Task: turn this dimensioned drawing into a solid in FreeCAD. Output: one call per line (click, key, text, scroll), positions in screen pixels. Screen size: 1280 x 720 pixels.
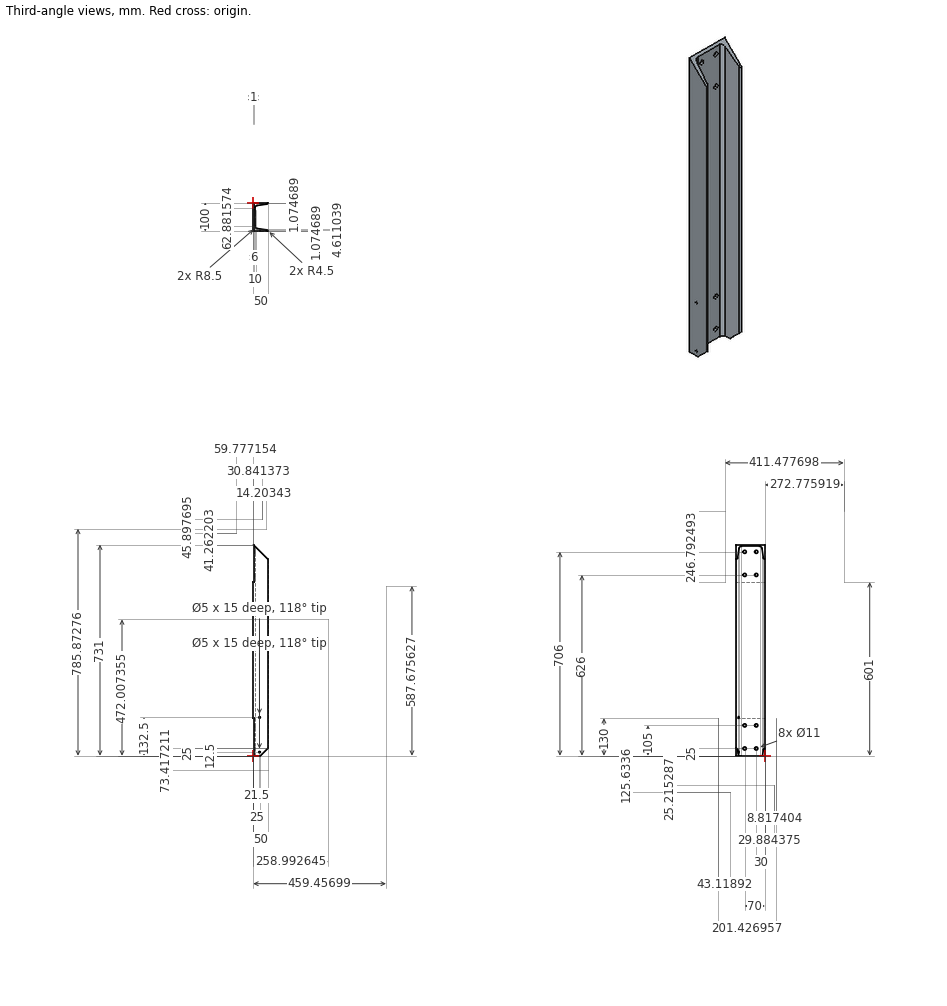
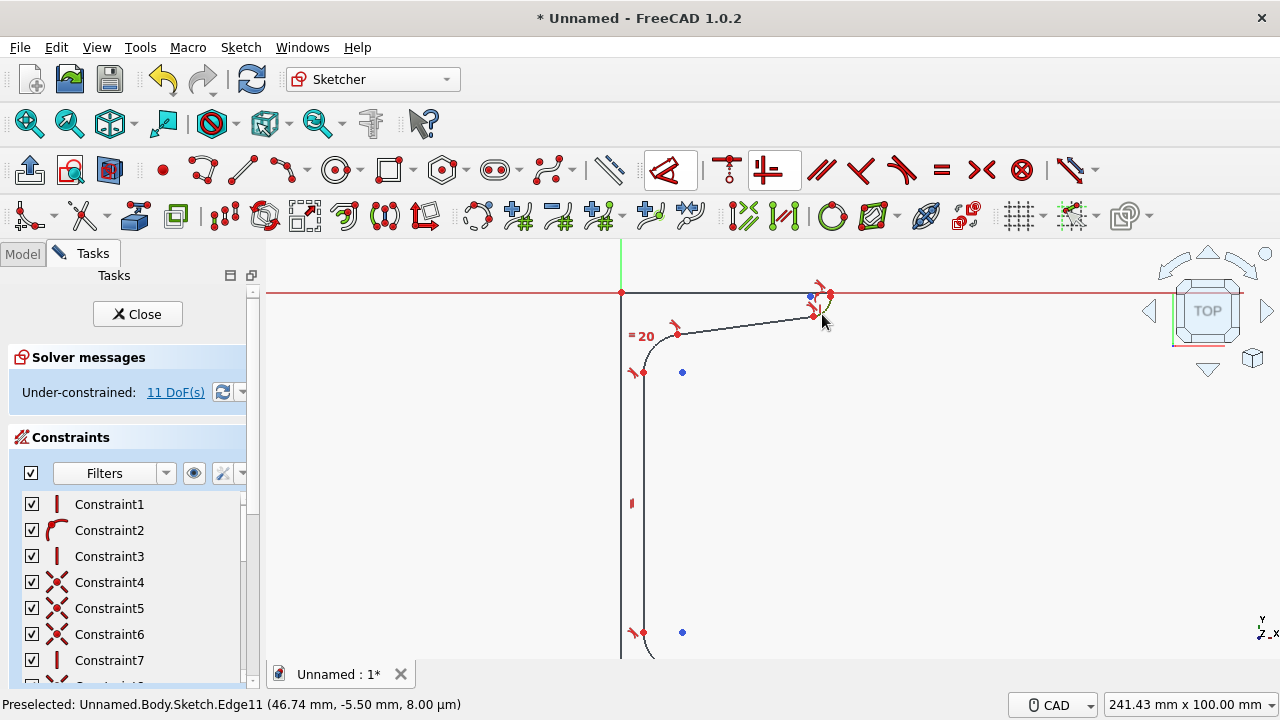
scroll(661, 340, down, 2)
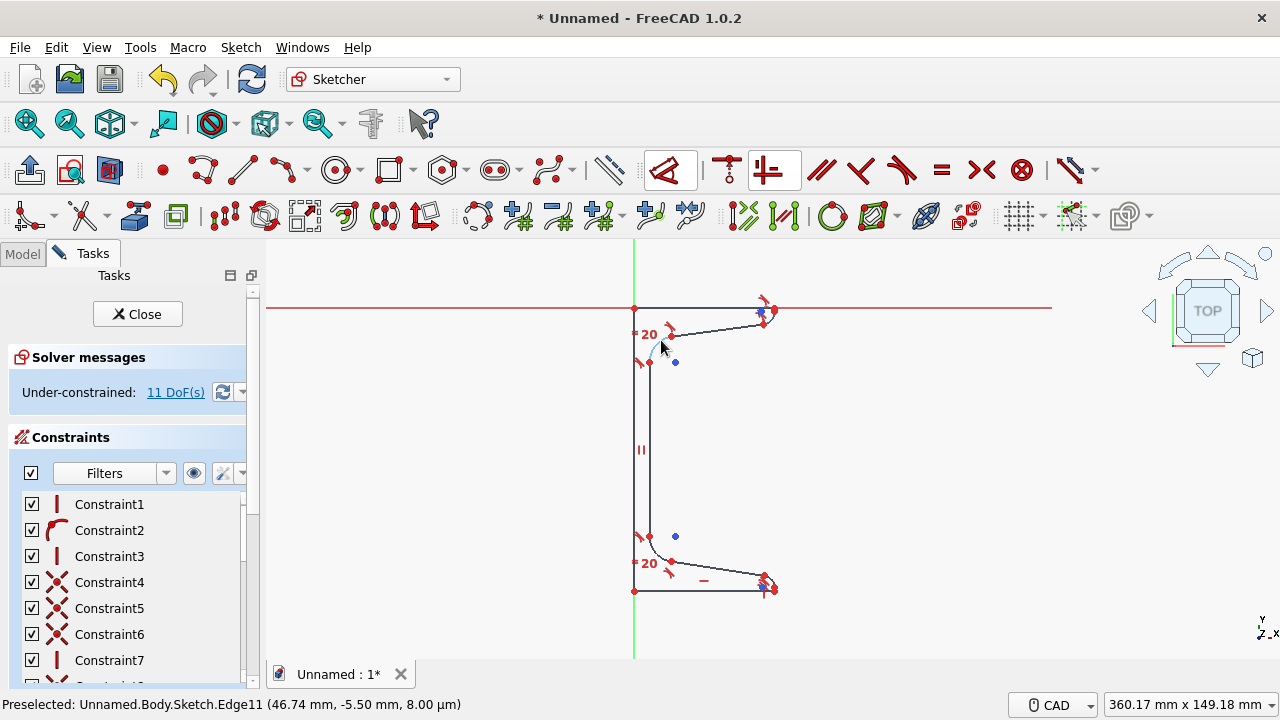
scroll(772, 580, up, 3)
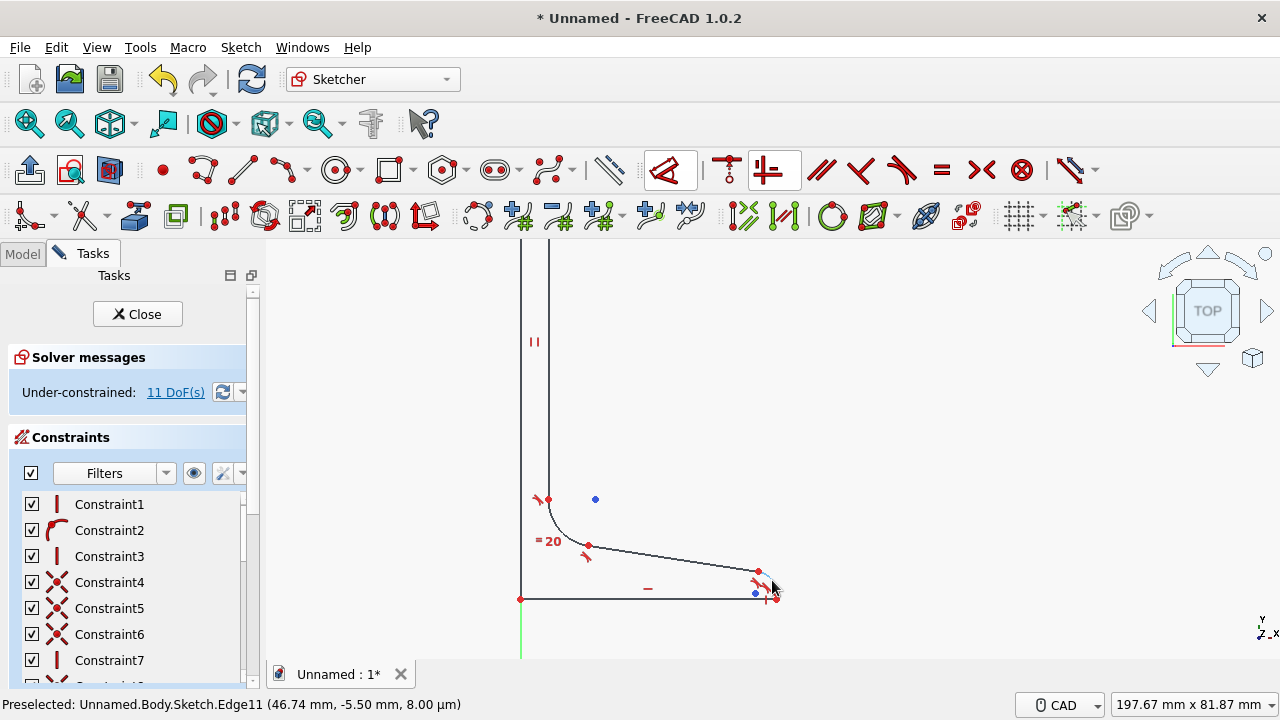
click(771, 579)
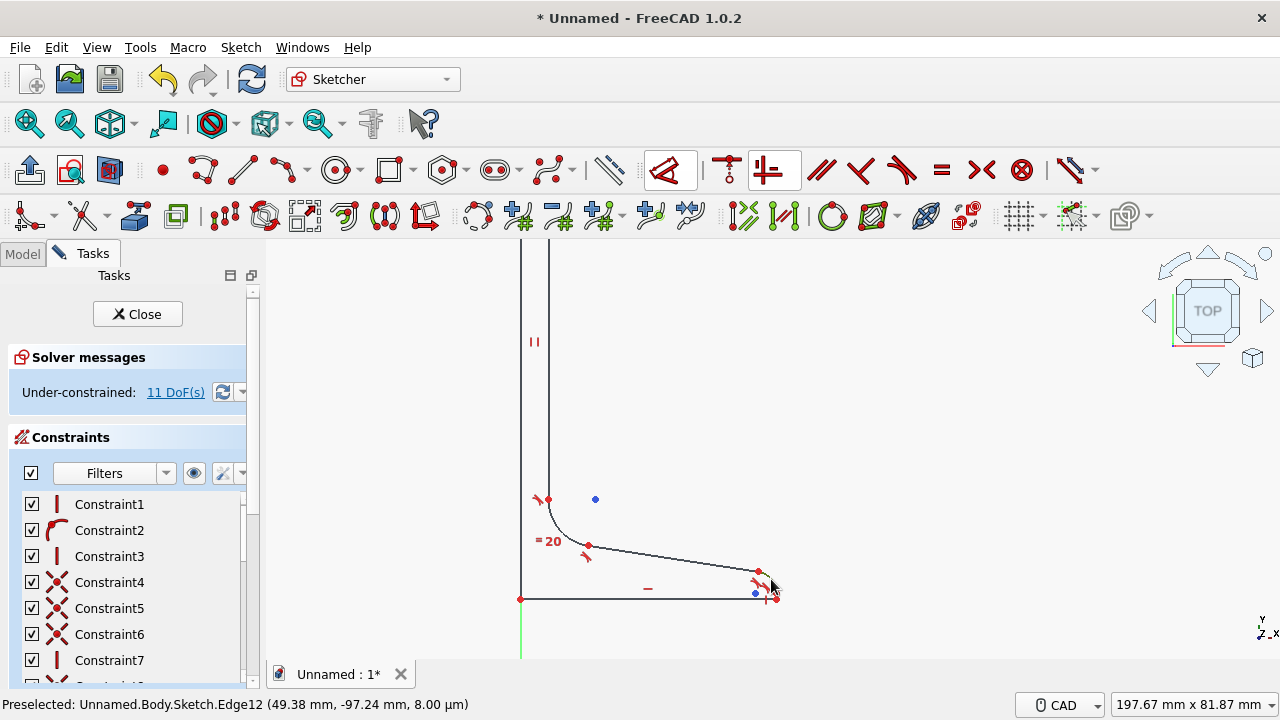
click(942, 170)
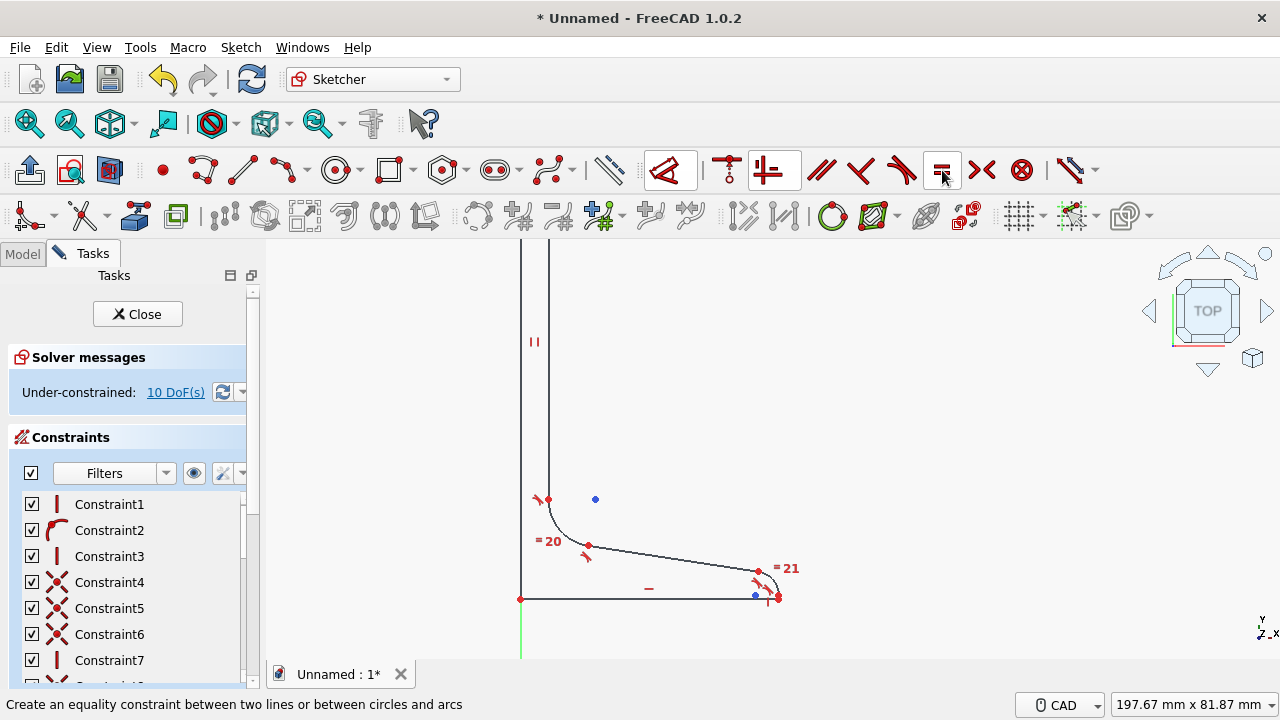
key(d)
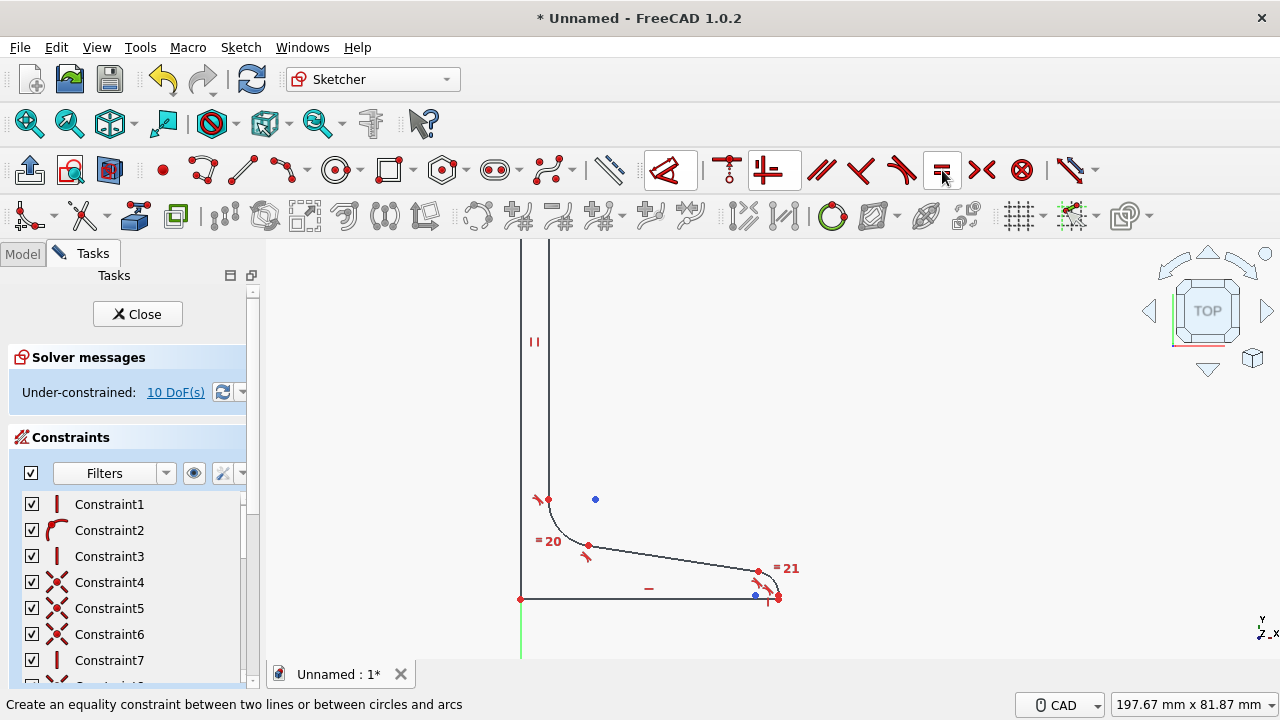
click(553, 519)
click(548, 563)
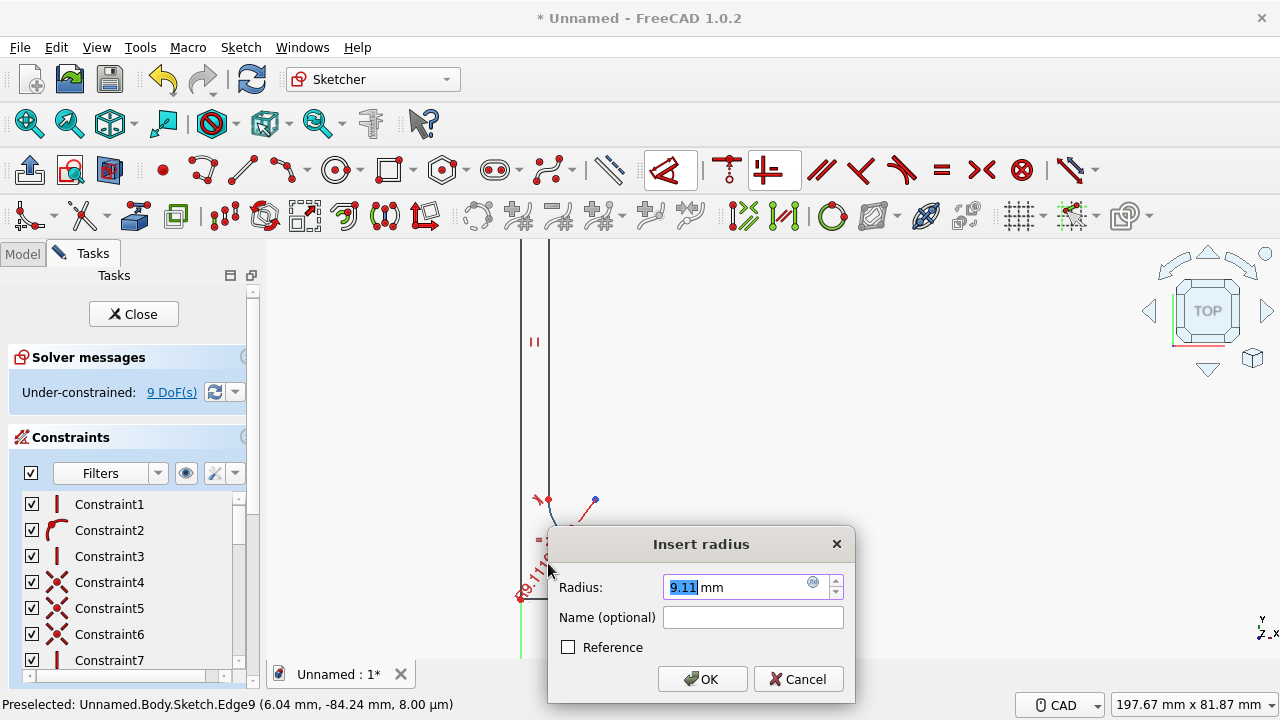
text(8.5)
key(Return)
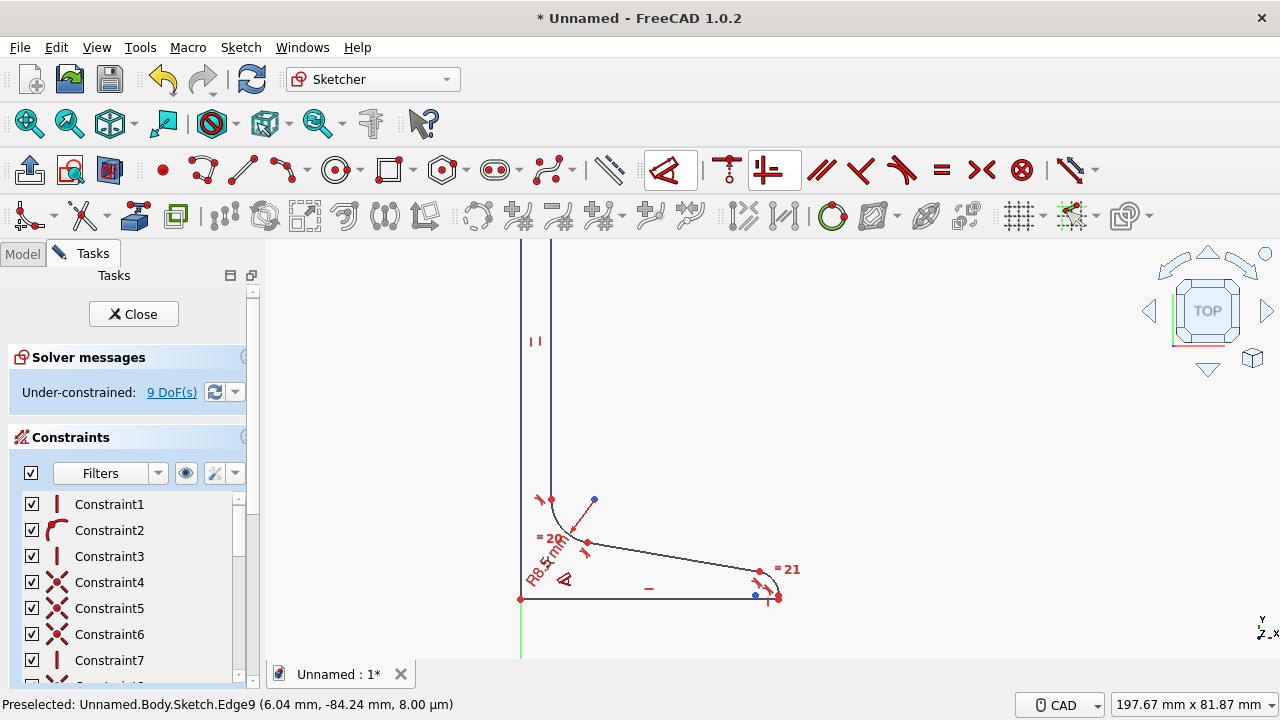
scroll(772, 581, down, 3)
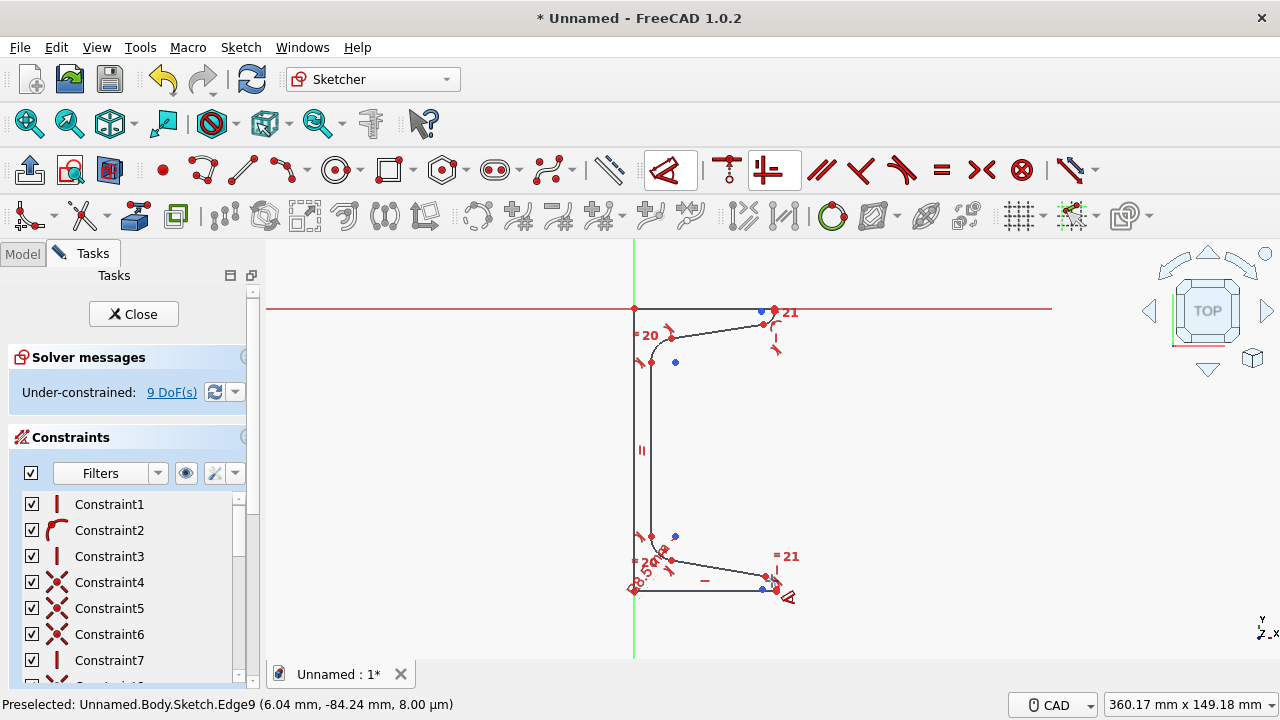
scroll(769, 323, up, 6)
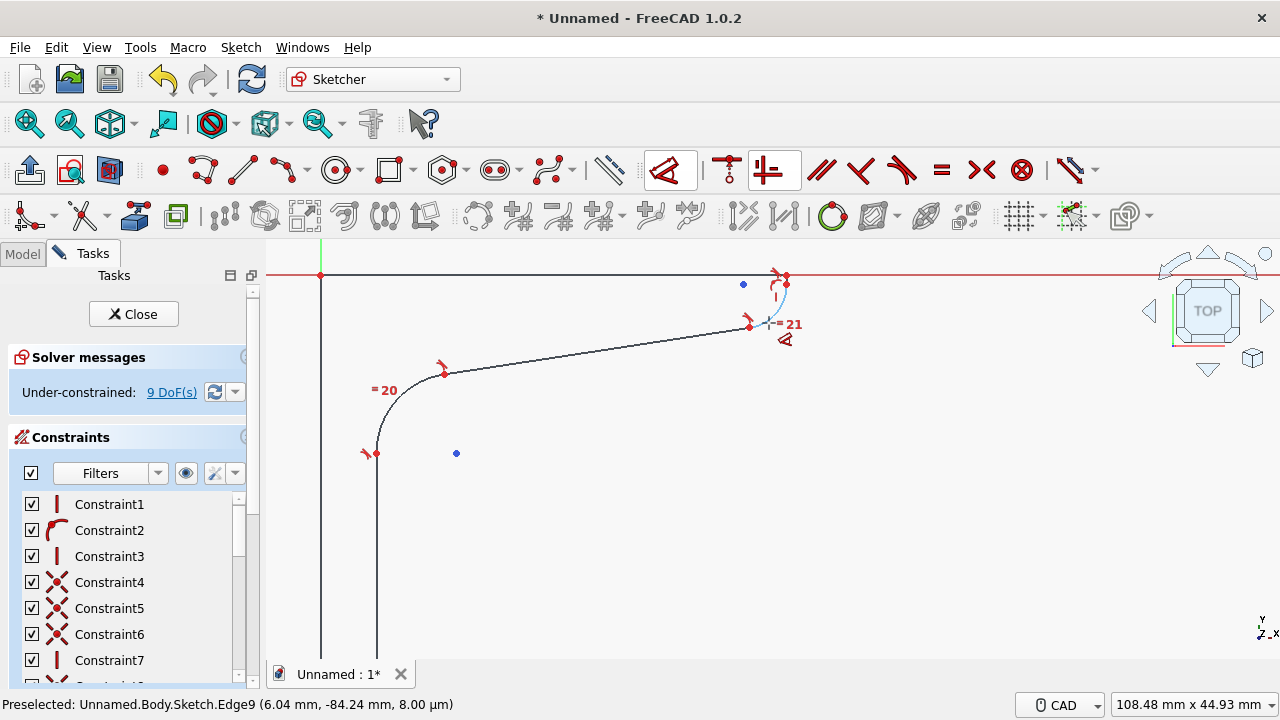
click(767, 321)
click(785, 348)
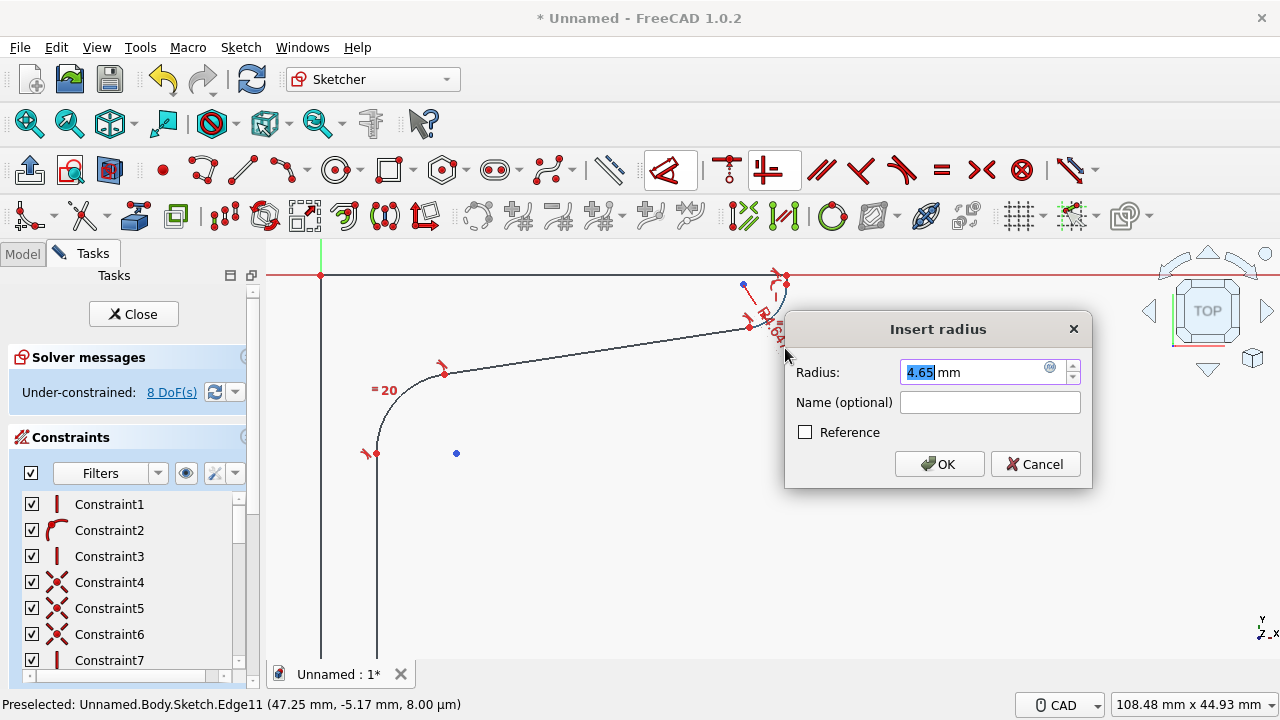
text(4.5)
key(Return)